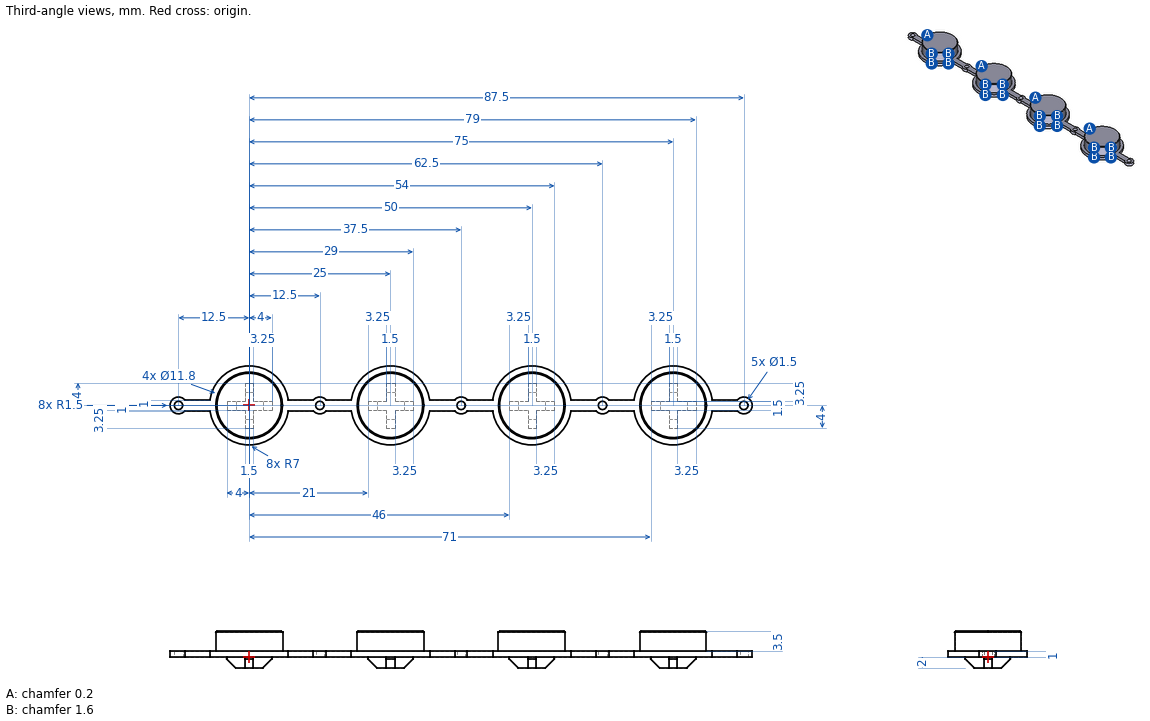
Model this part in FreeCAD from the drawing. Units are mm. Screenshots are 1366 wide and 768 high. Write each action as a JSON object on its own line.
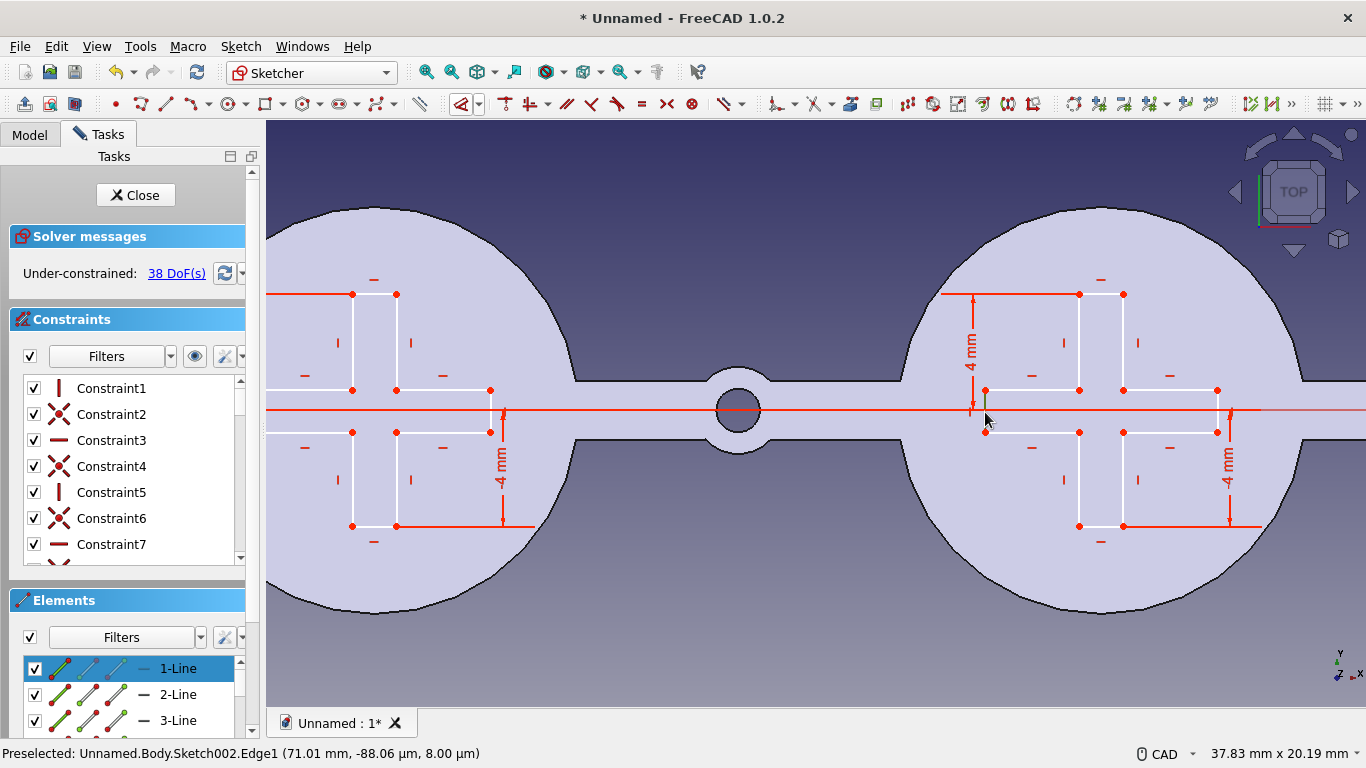
{"action": "key", "text": "i"}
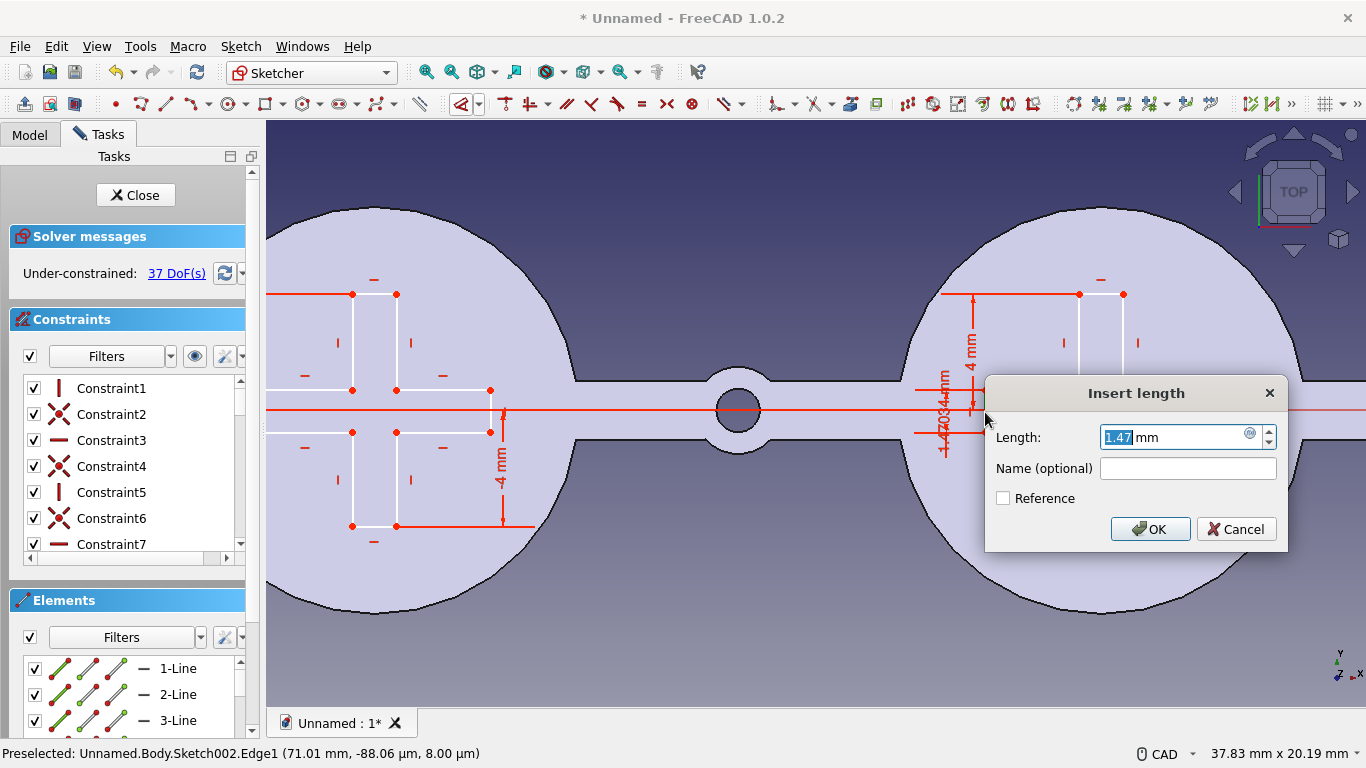
{"action": "type", "text": "1.5"}
{"action": "key", "text": "Return"}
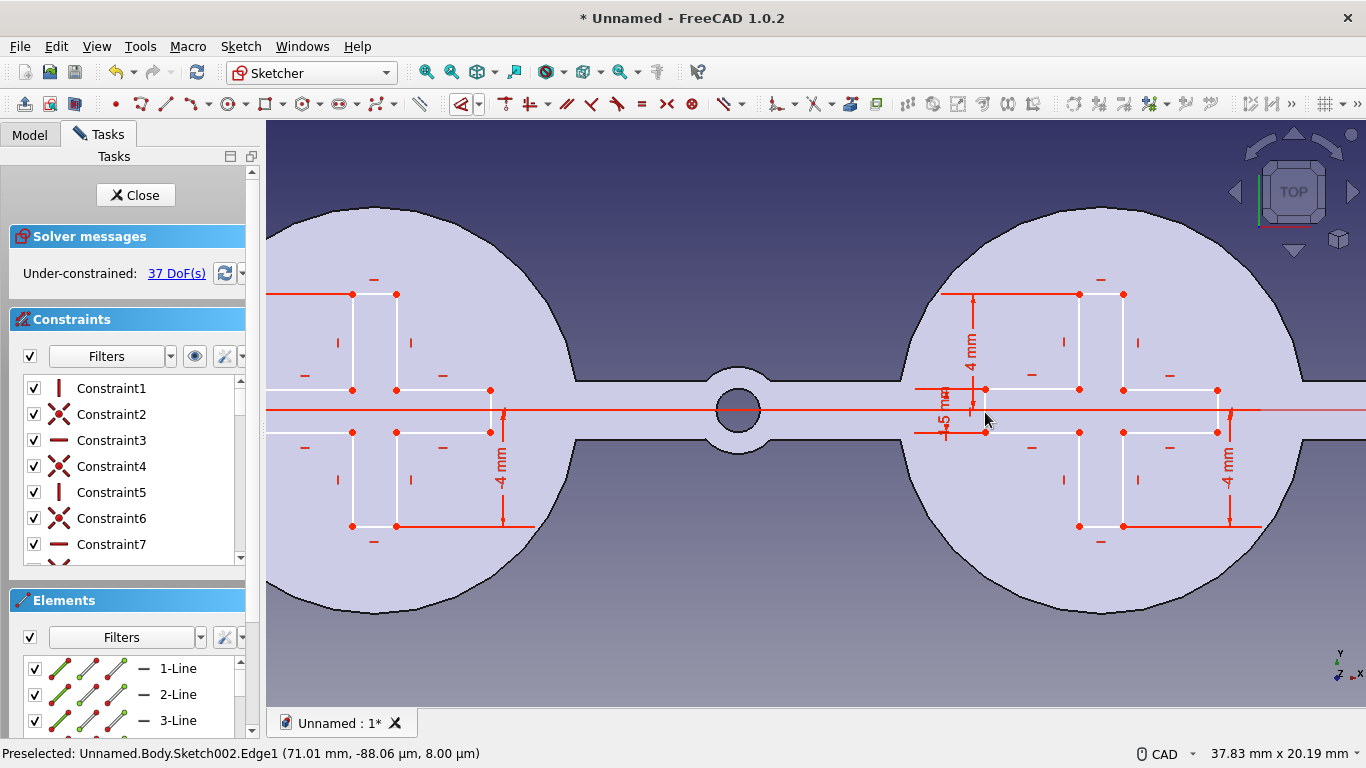
{"action": "left_click", "coordinate": [1093, 294]}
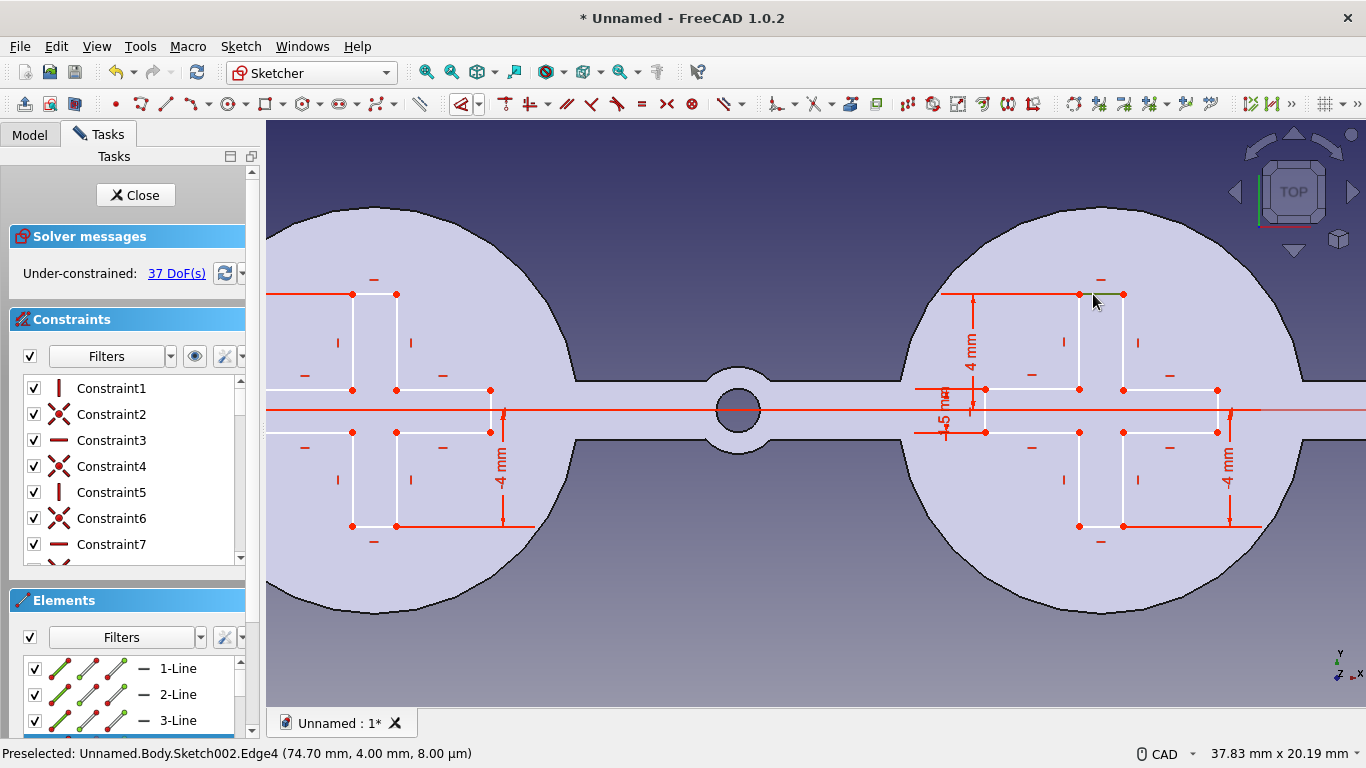
{"action": "key", "text": "l"}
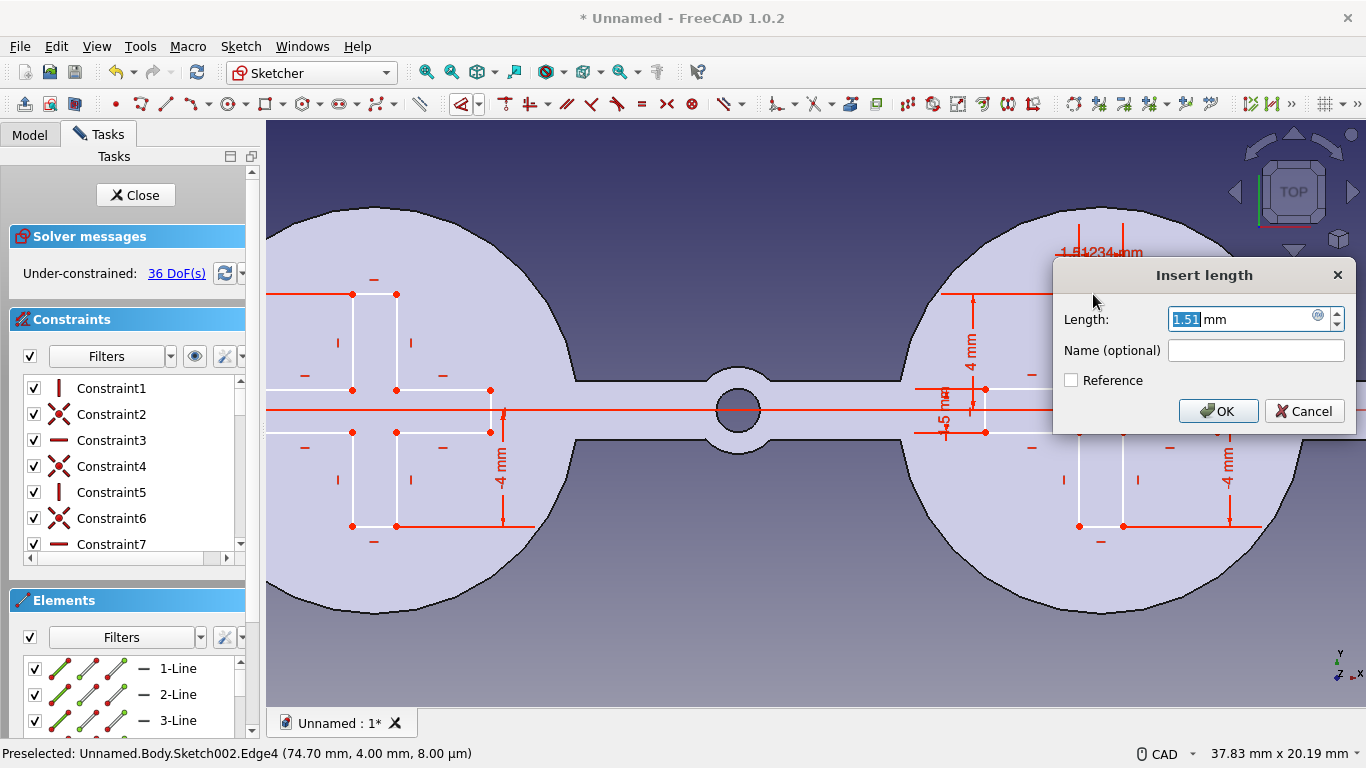
{"action": "type", "text": "1.5"}
{"action": "key", "text": "Return"}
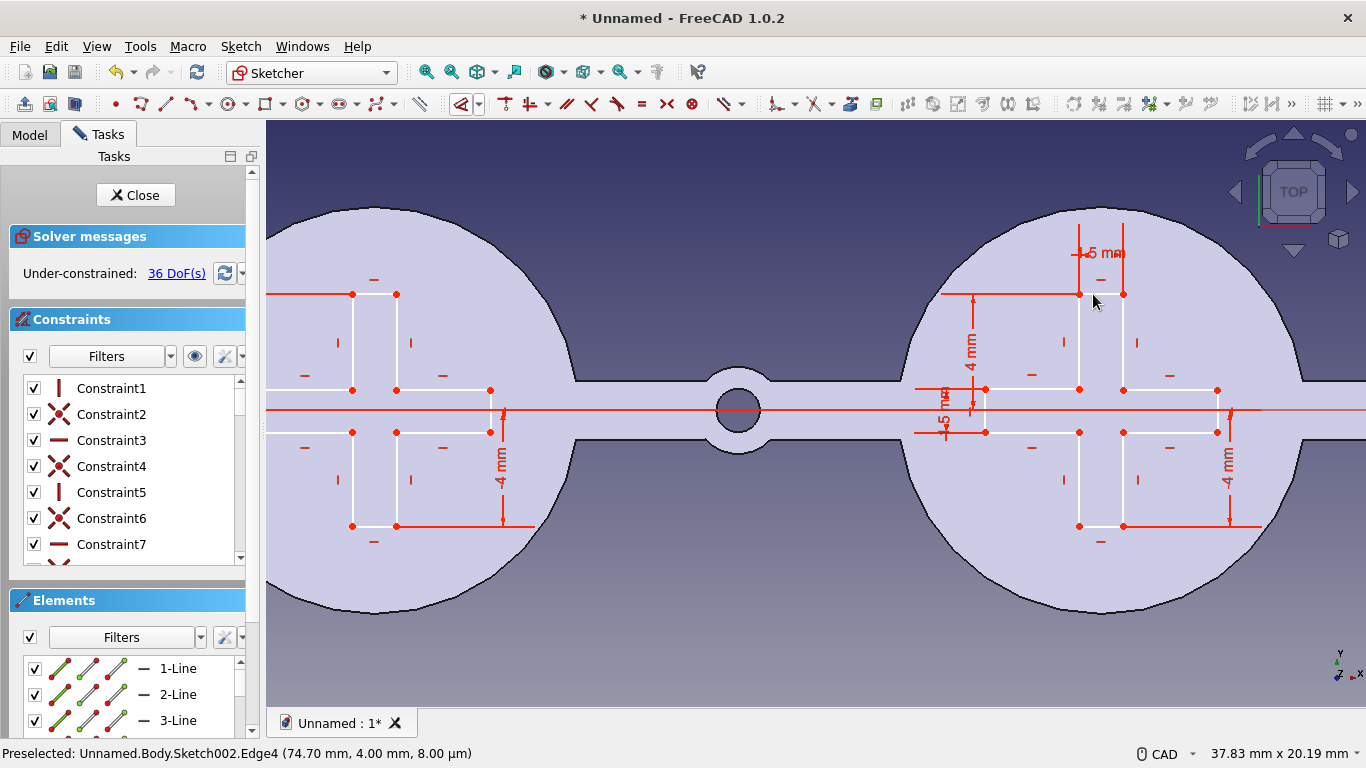
{"action": "scroll", "coordinate": [988, 415], "scroll_direction": "down", "scroll_amount": 7}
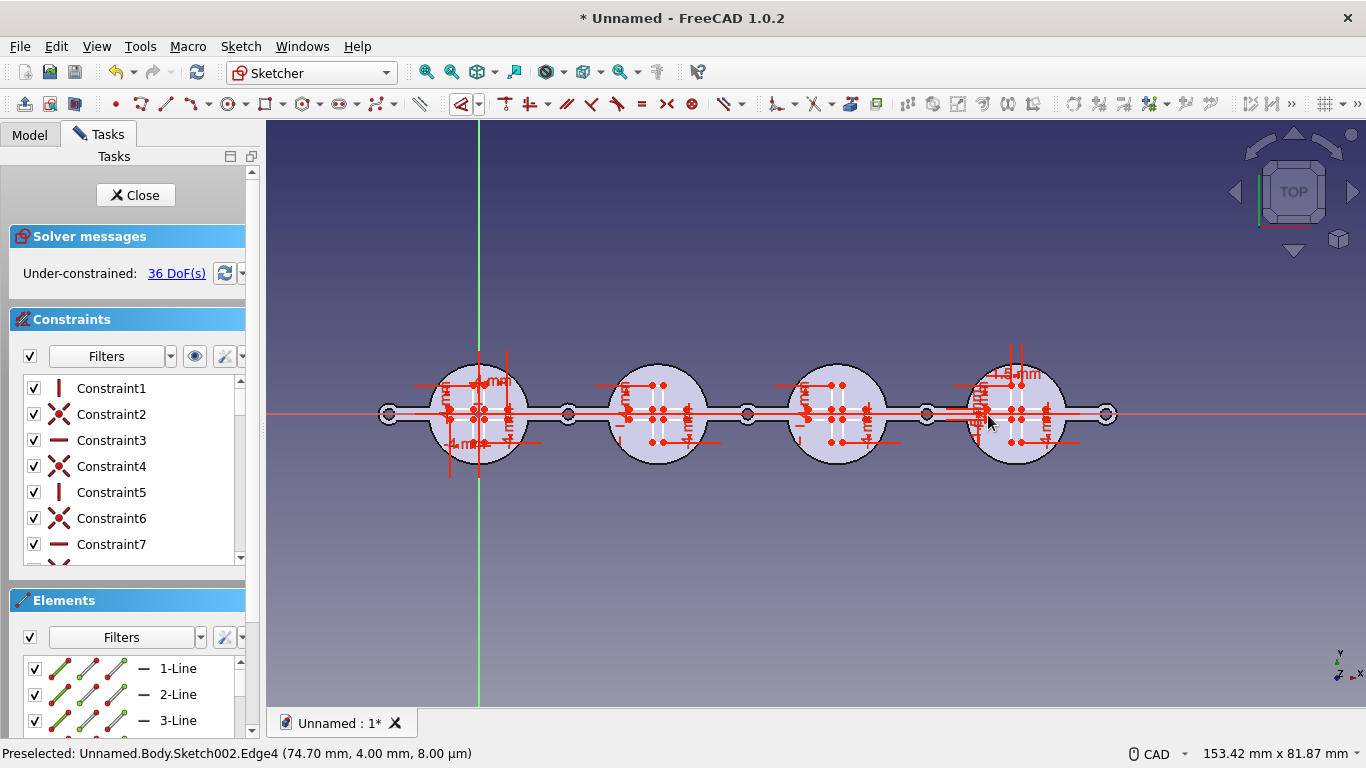
{"action": "scroll", "coordinate": [1045, 417], "scroll_direction": "up", "scroll_amount": 9}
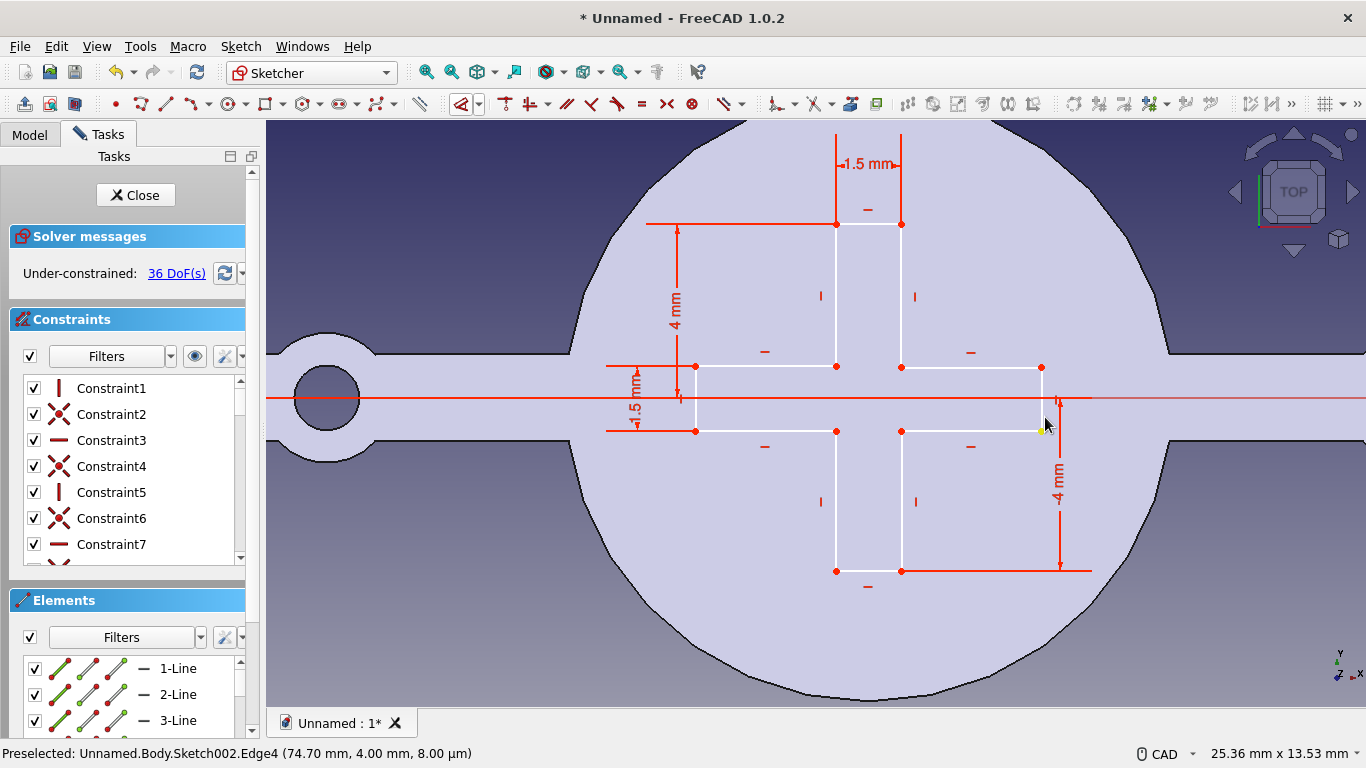
{"action": "left_click", "coordinate": [1042, 412]}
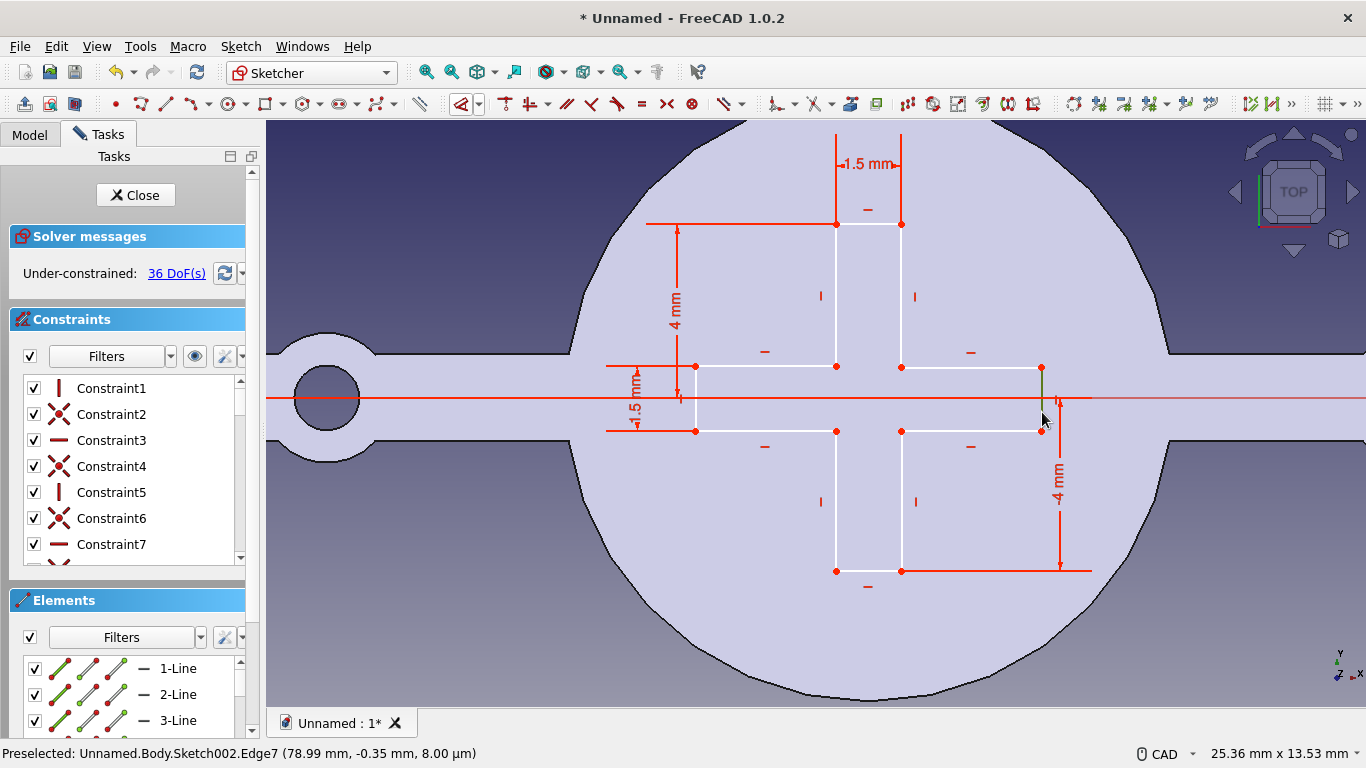
{"action": "key", "text": "i"}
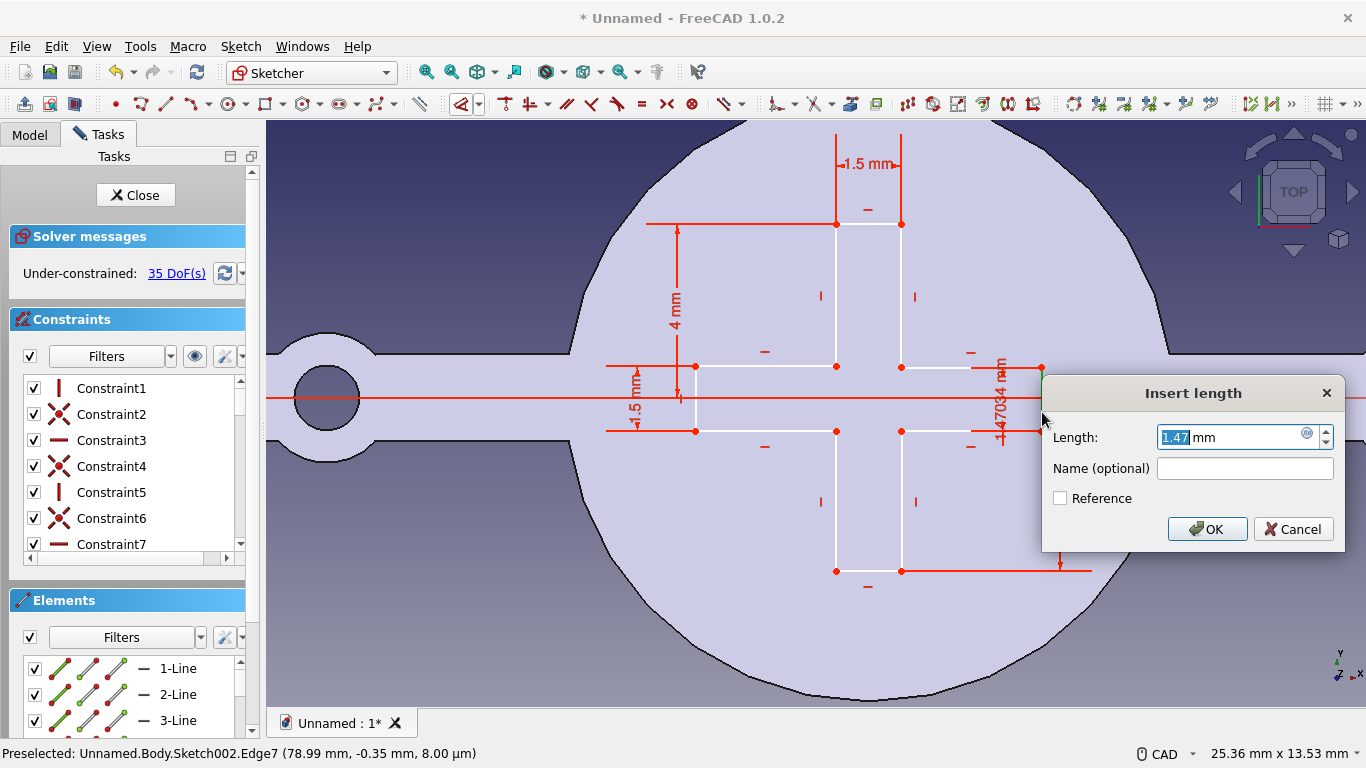
{"action": "type", "text": "1.5"}
{"action": "key", "text": "Return"}